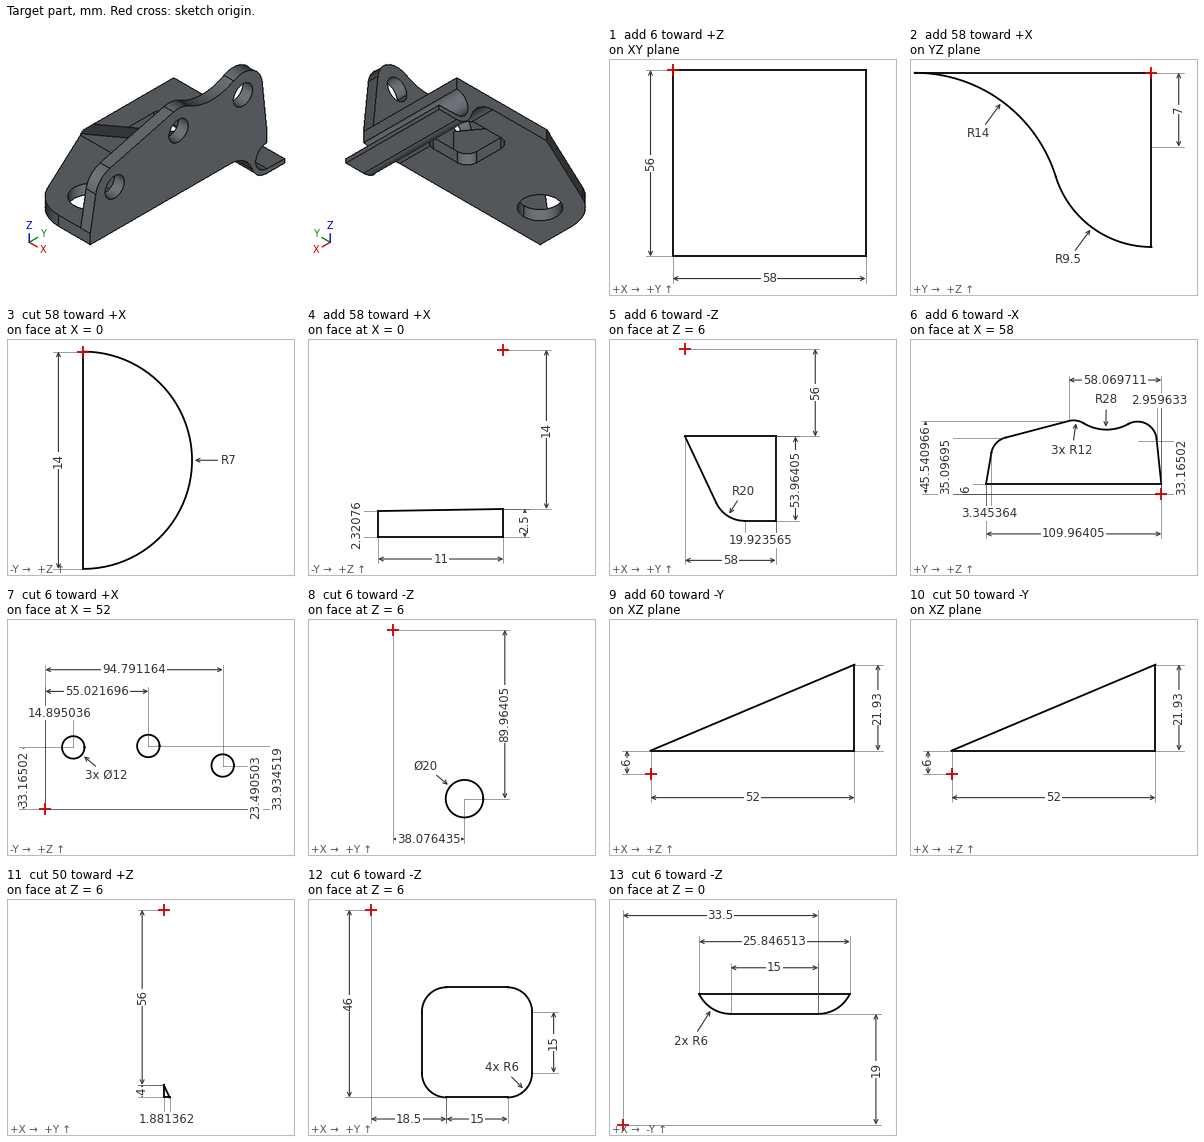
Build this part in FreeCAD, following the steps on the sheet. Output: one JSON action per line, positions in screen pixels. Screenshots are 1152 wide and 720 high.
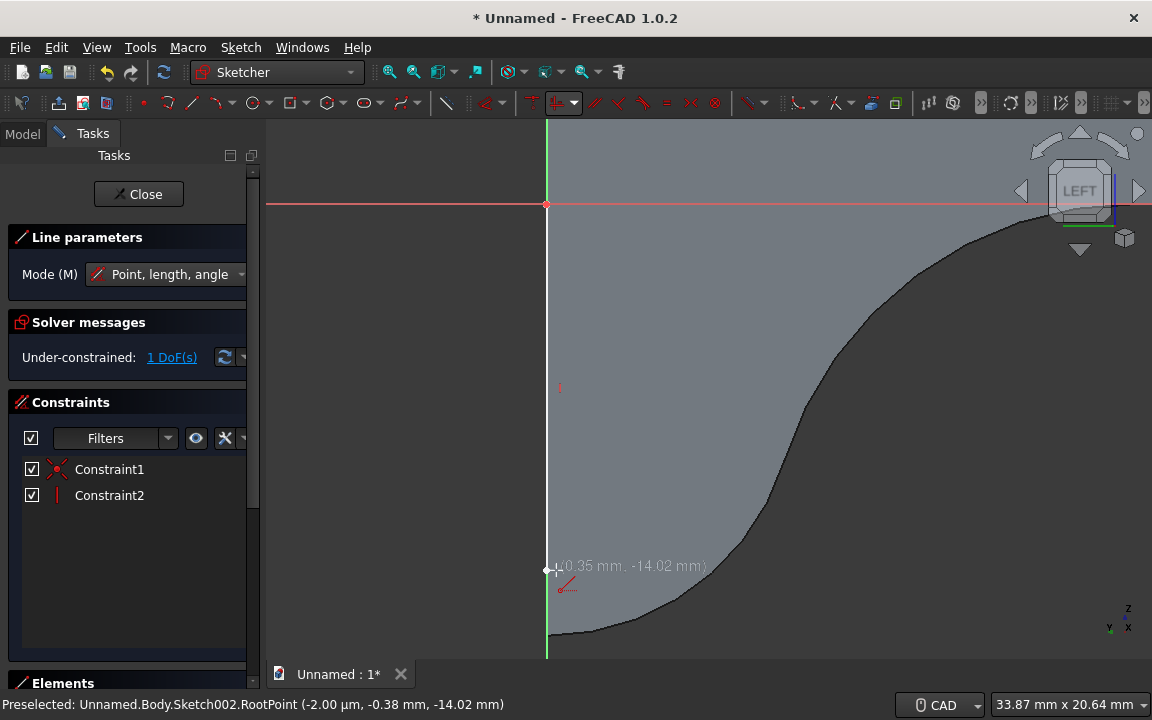
{"action": "left_click", "coordinate": [216, 104]}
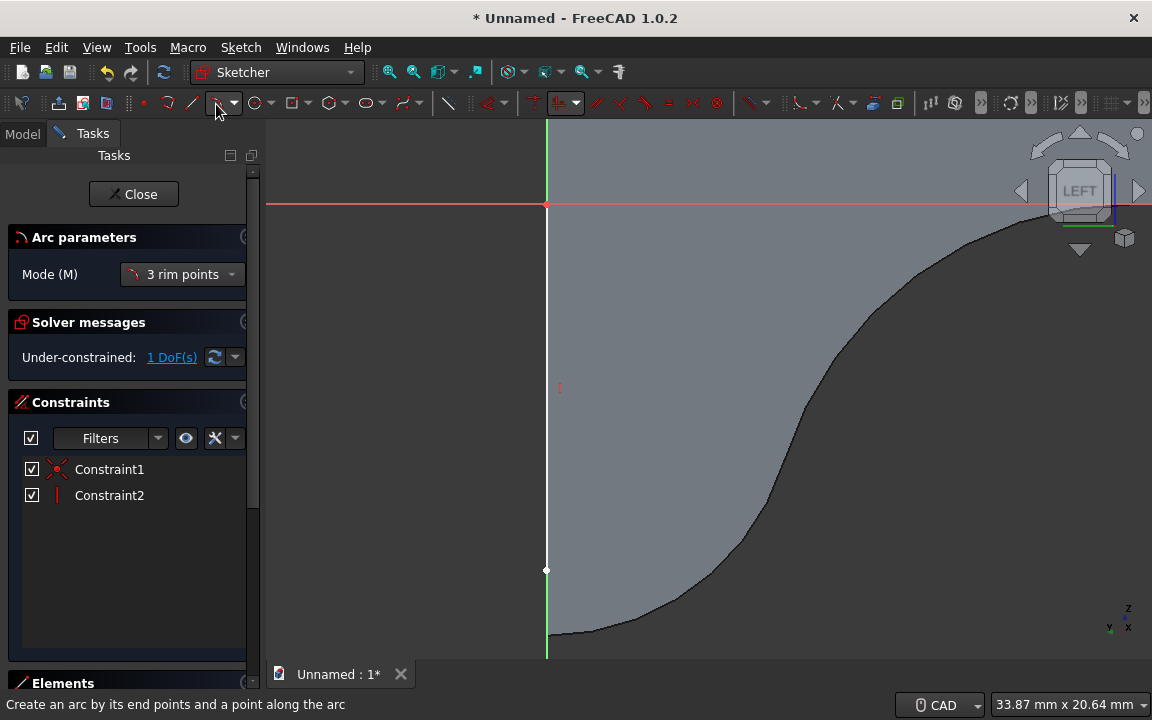
{"action": "left_click", "coordinate": [556, 570]}
{"action": "left_click", "coordinate": [547, 204]}
{"action": "left_click", "coordinate": [730, 387]}
{"action": "key", "text": "Escape"}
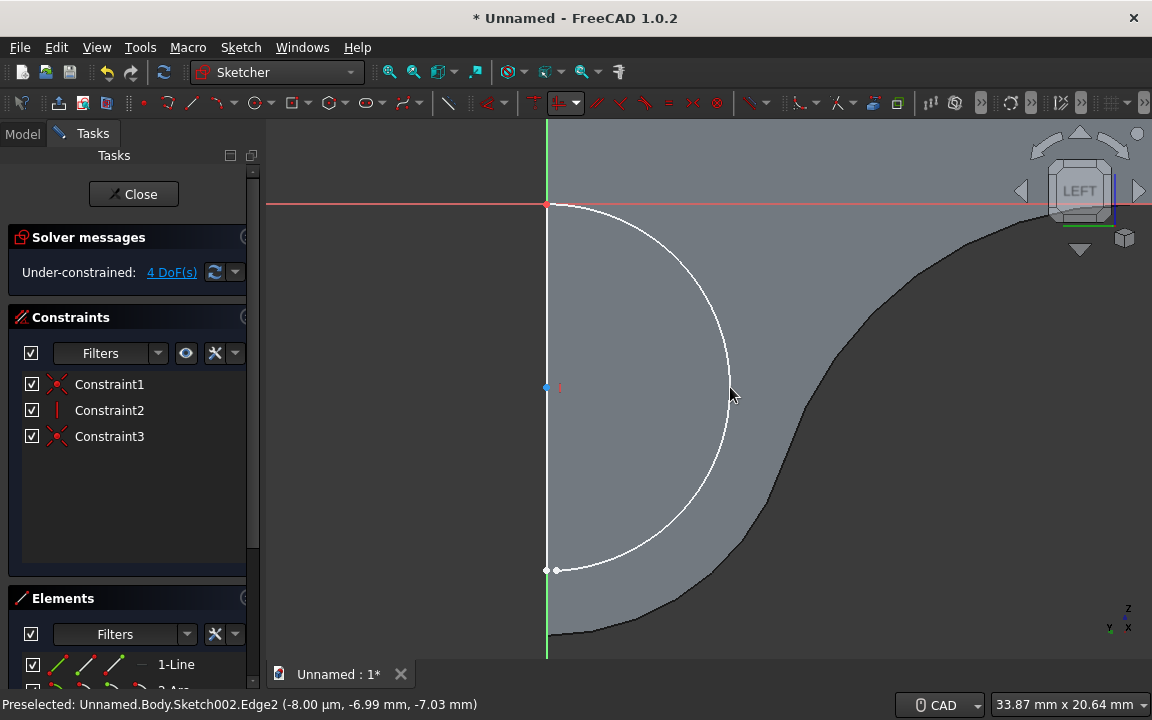
{"action": "left_click", "coordinate": [546, 388]}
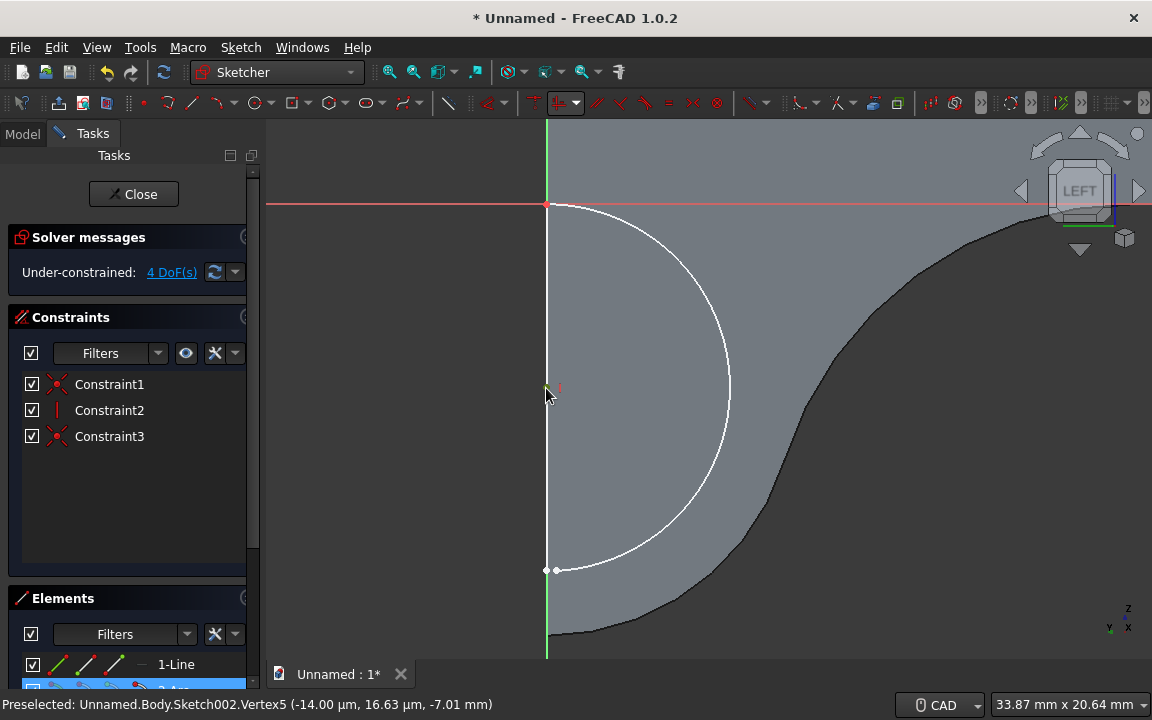
{"action": "left_click", "coordinate": [547, 596]}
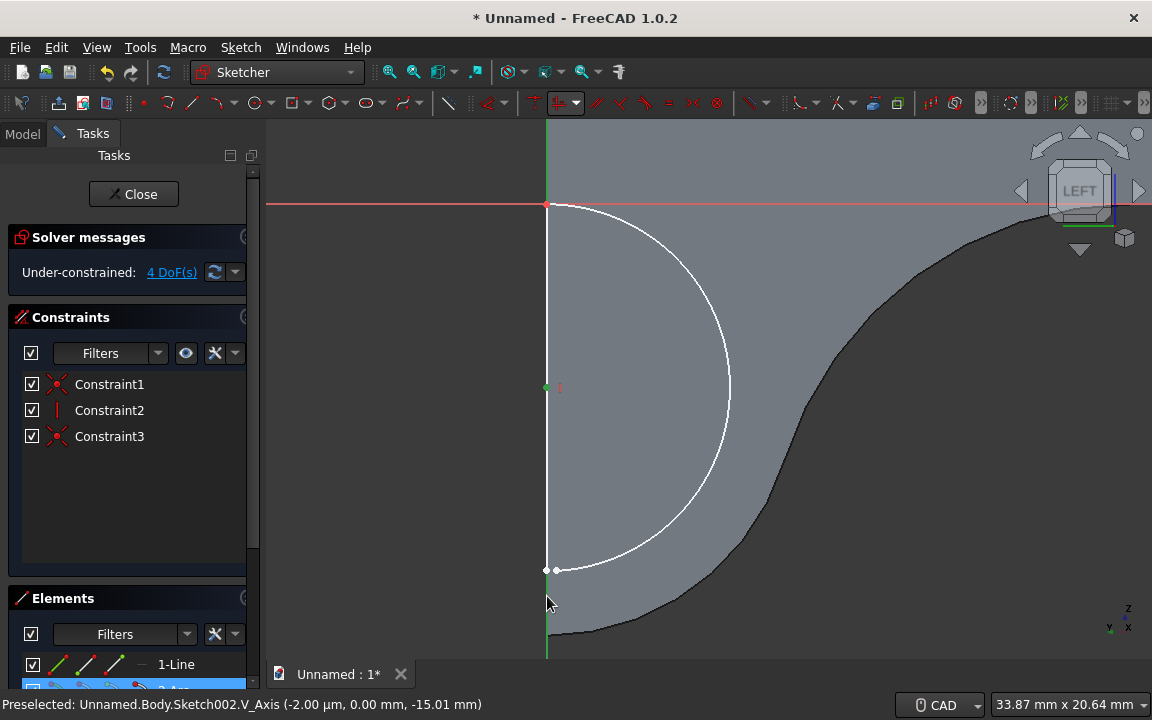
{"action": "left_click", "coordinate": [534, 104]}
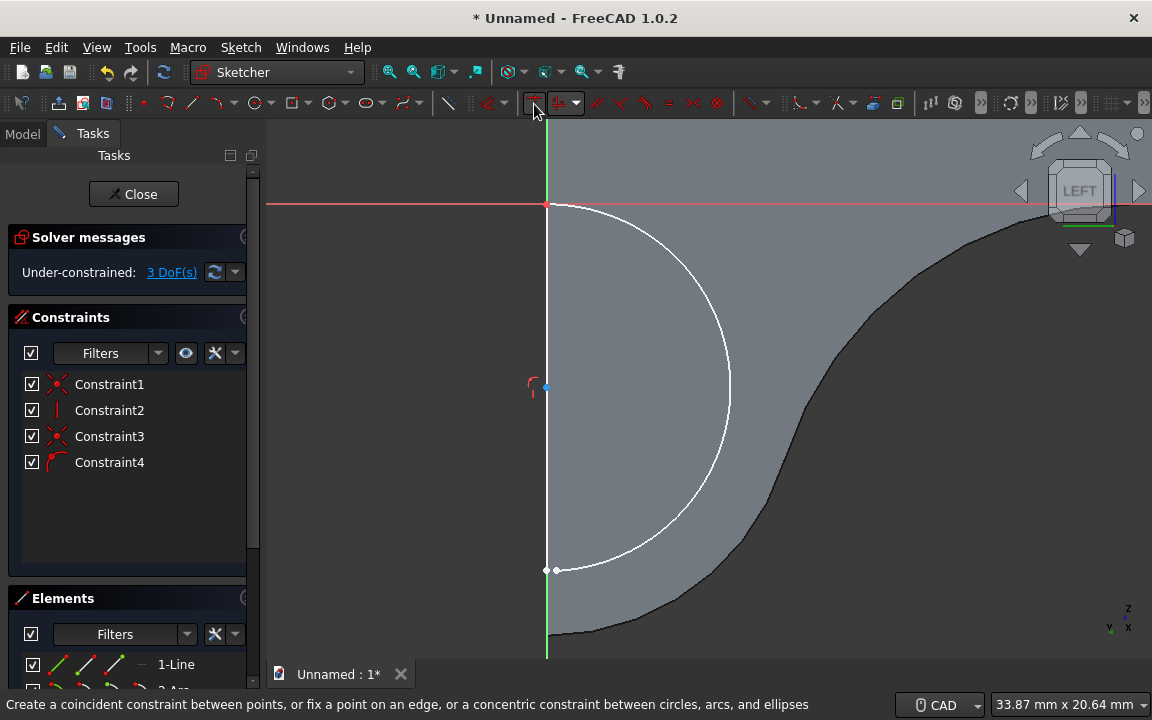
{"action": "left_click", "coordinate": [488, 104]}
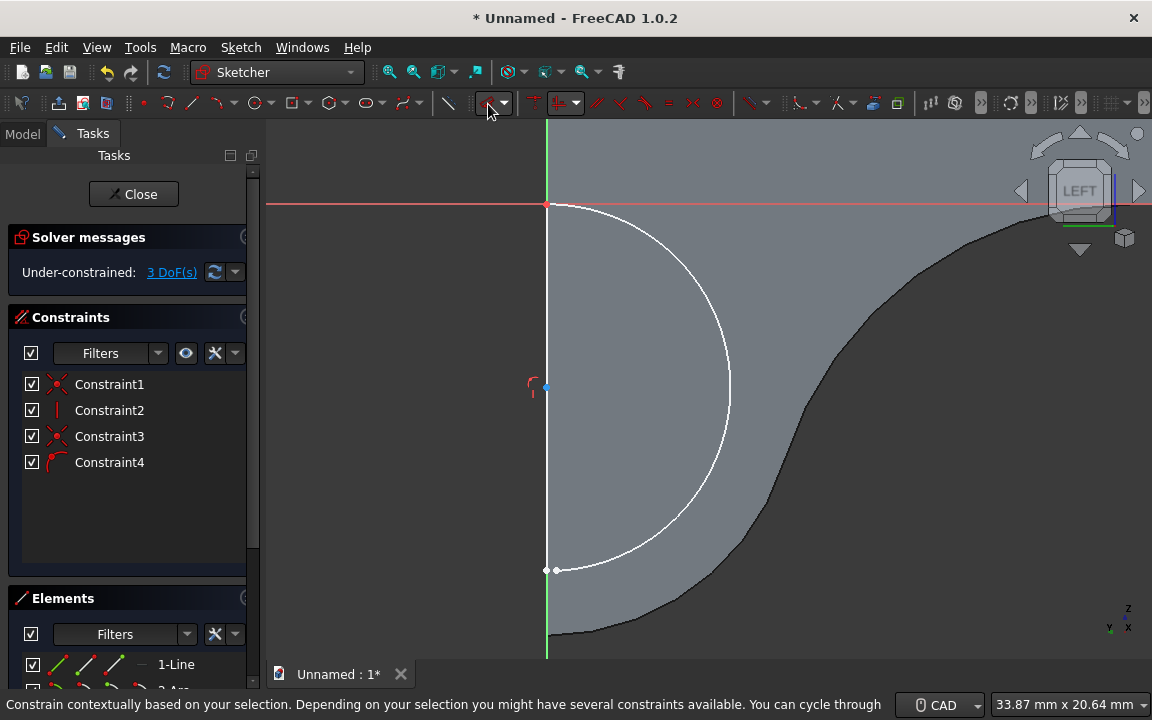
{"action": "left_click", "coordinate": [699, 490]}
{"action": "left_click", "coordinate": [726, 508]}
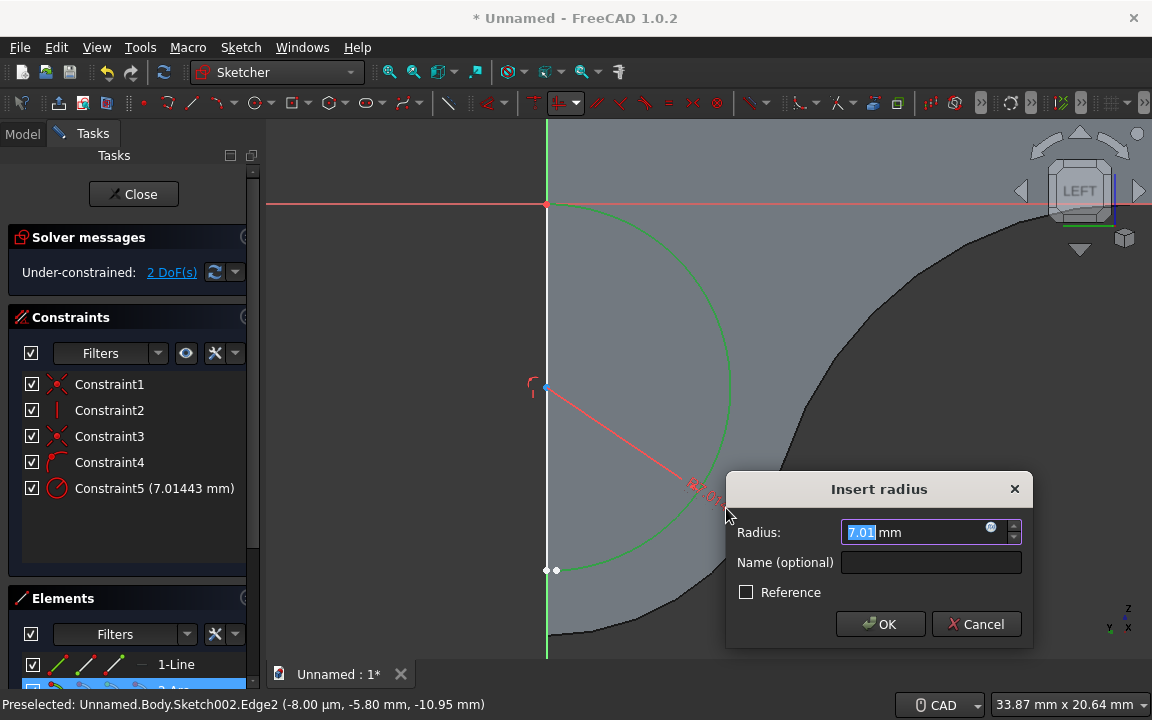
{"action": "type", "text": "7"}
{"action": "key", "text": "Return"}
{"action": "key", "text": "Escape"}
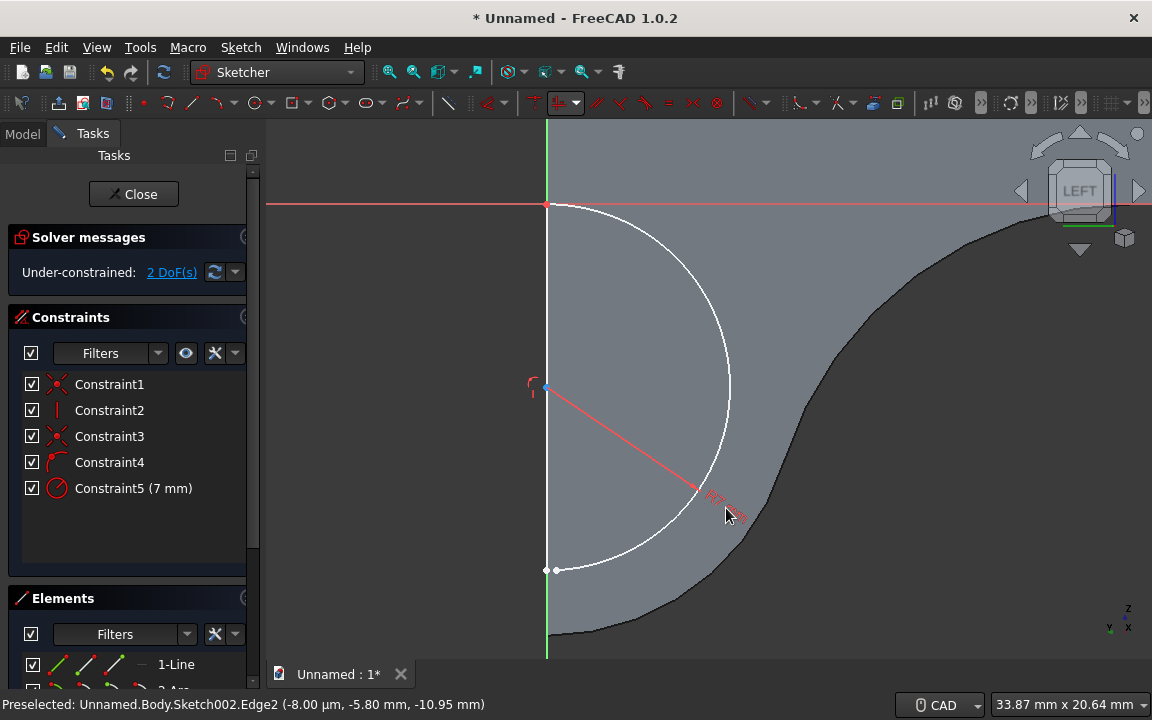
{"action": "left_click", "coordinate": [556, 570]}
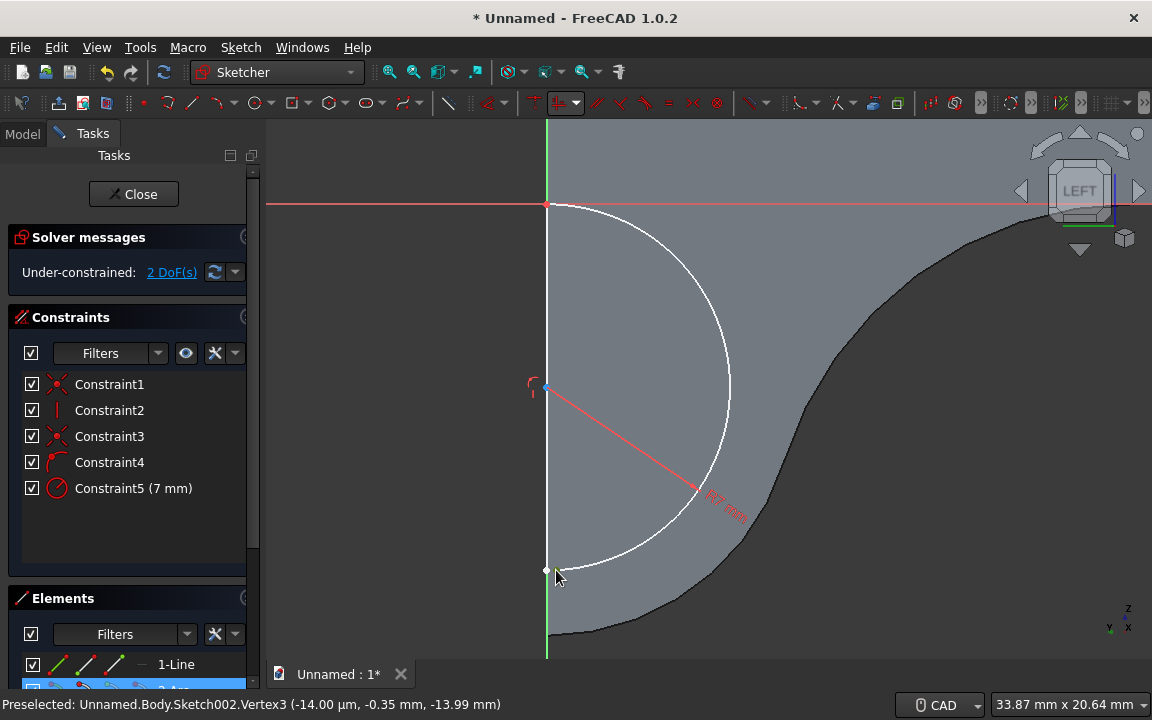
{"action": "left_click", "coordinate": [547, 596]}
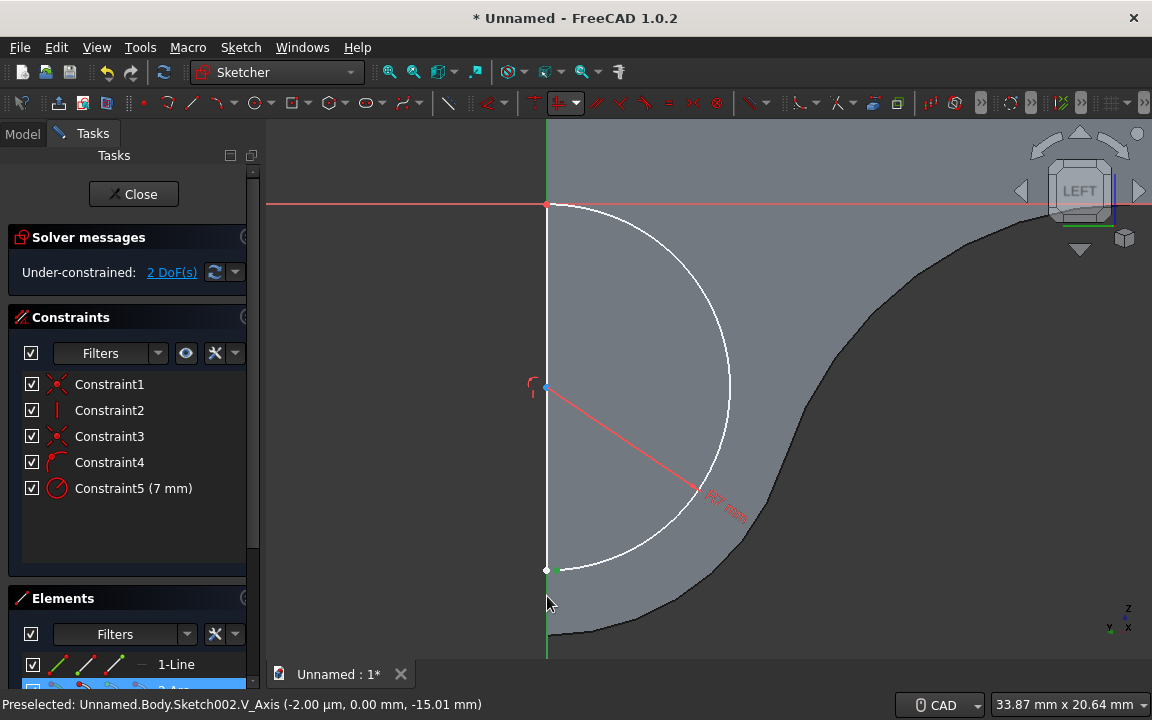
{"action": "key", "text": "c"}